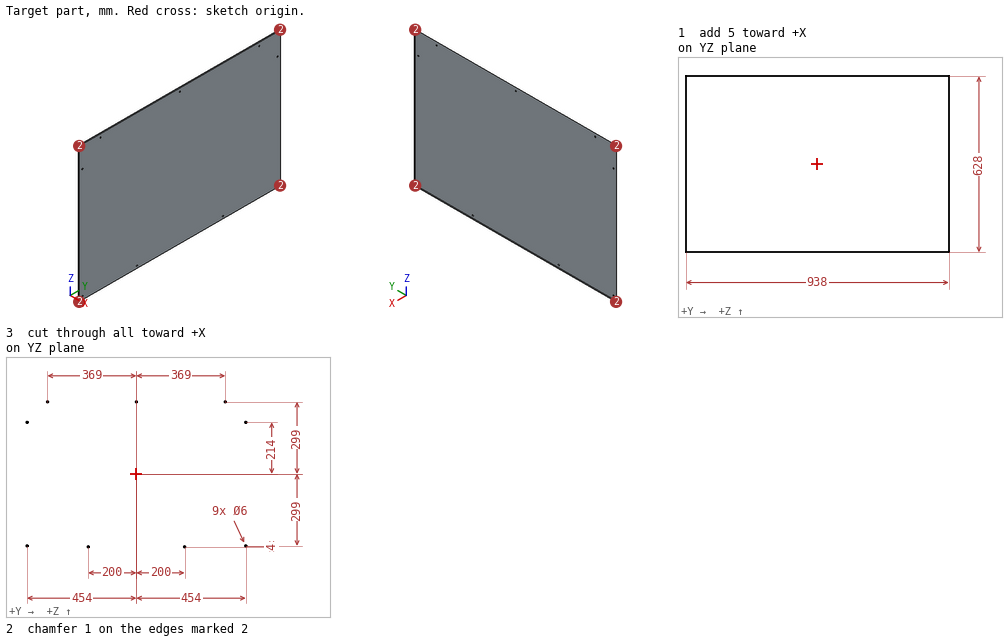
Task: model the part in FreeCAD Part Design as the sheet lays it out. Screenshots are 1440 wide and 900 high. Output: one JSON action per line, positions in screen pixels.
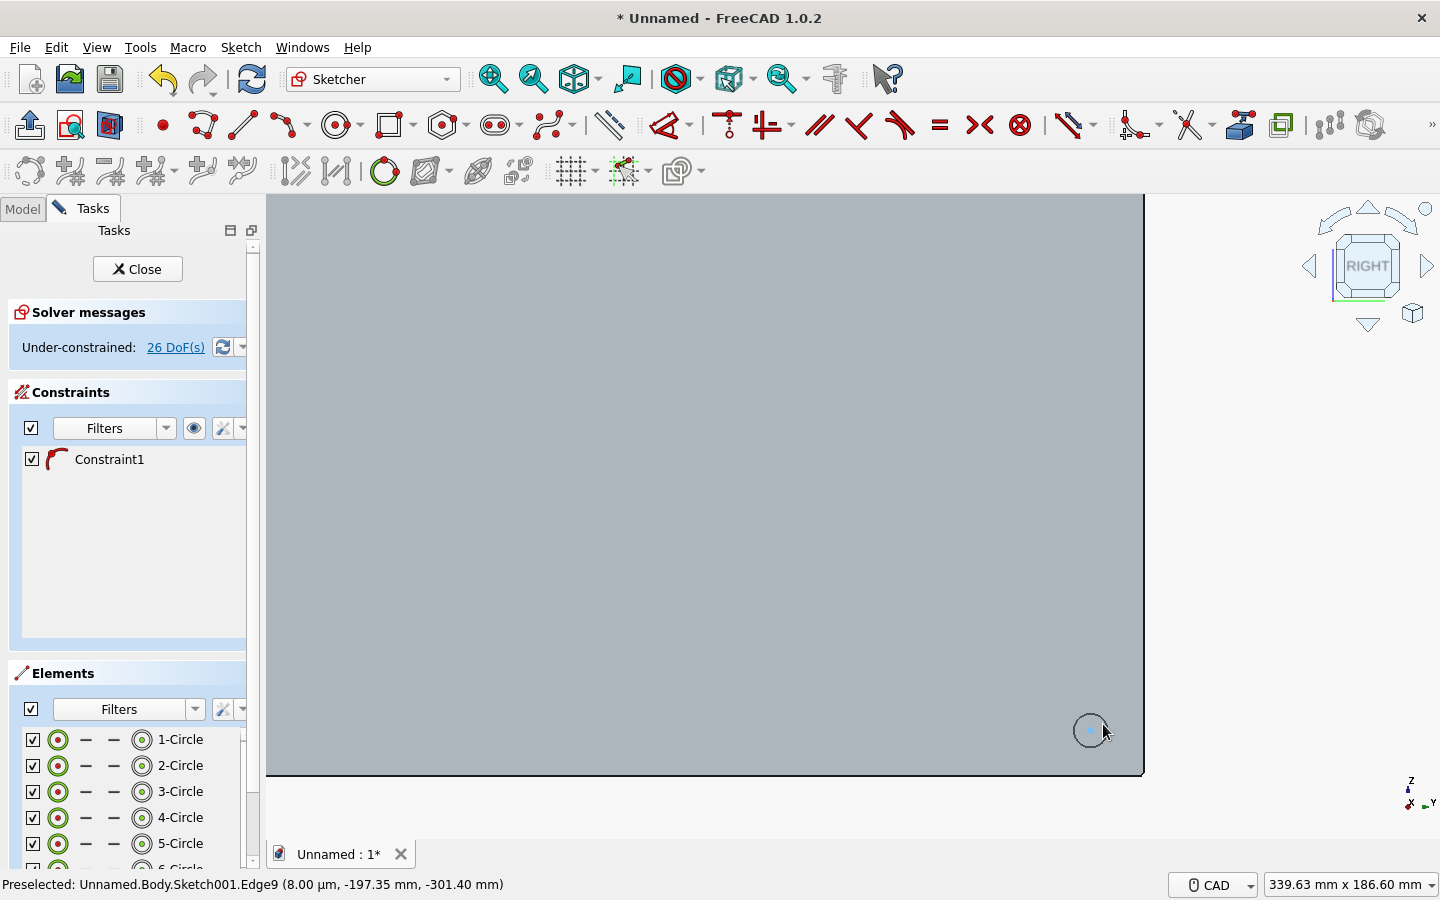
{"action": "left_click", "coordinate": [1103, 719]}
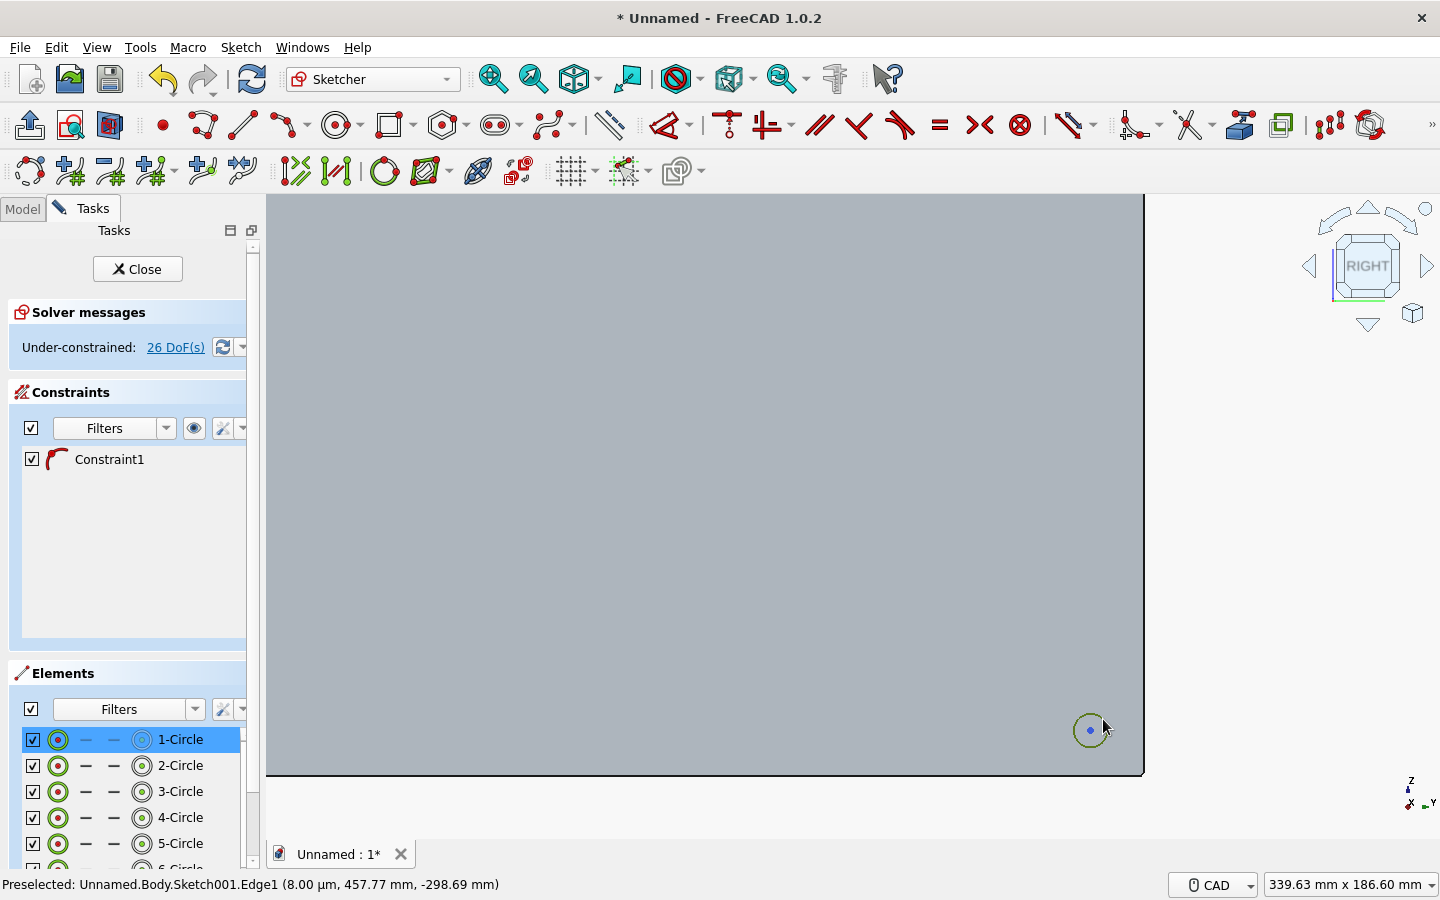
{"action": "scroll", "coordinate": [1104, 724], "scroll_direction": "down", "scroll_amount": 8}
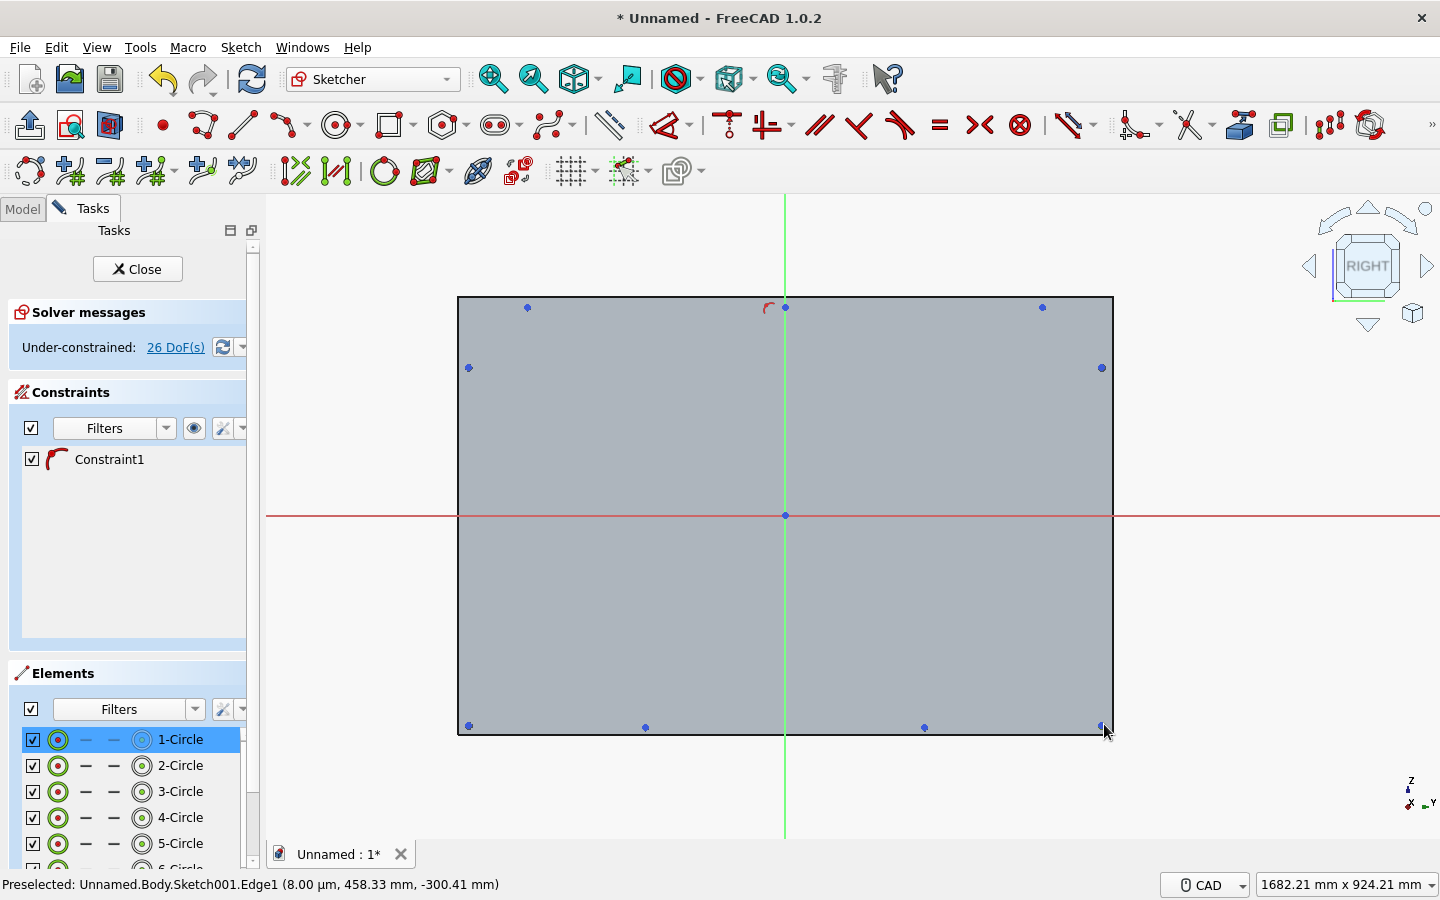
{"action": "scroll", "coordinate": [471, 724], "scroll_direction": "up", "scroll_amount": 8}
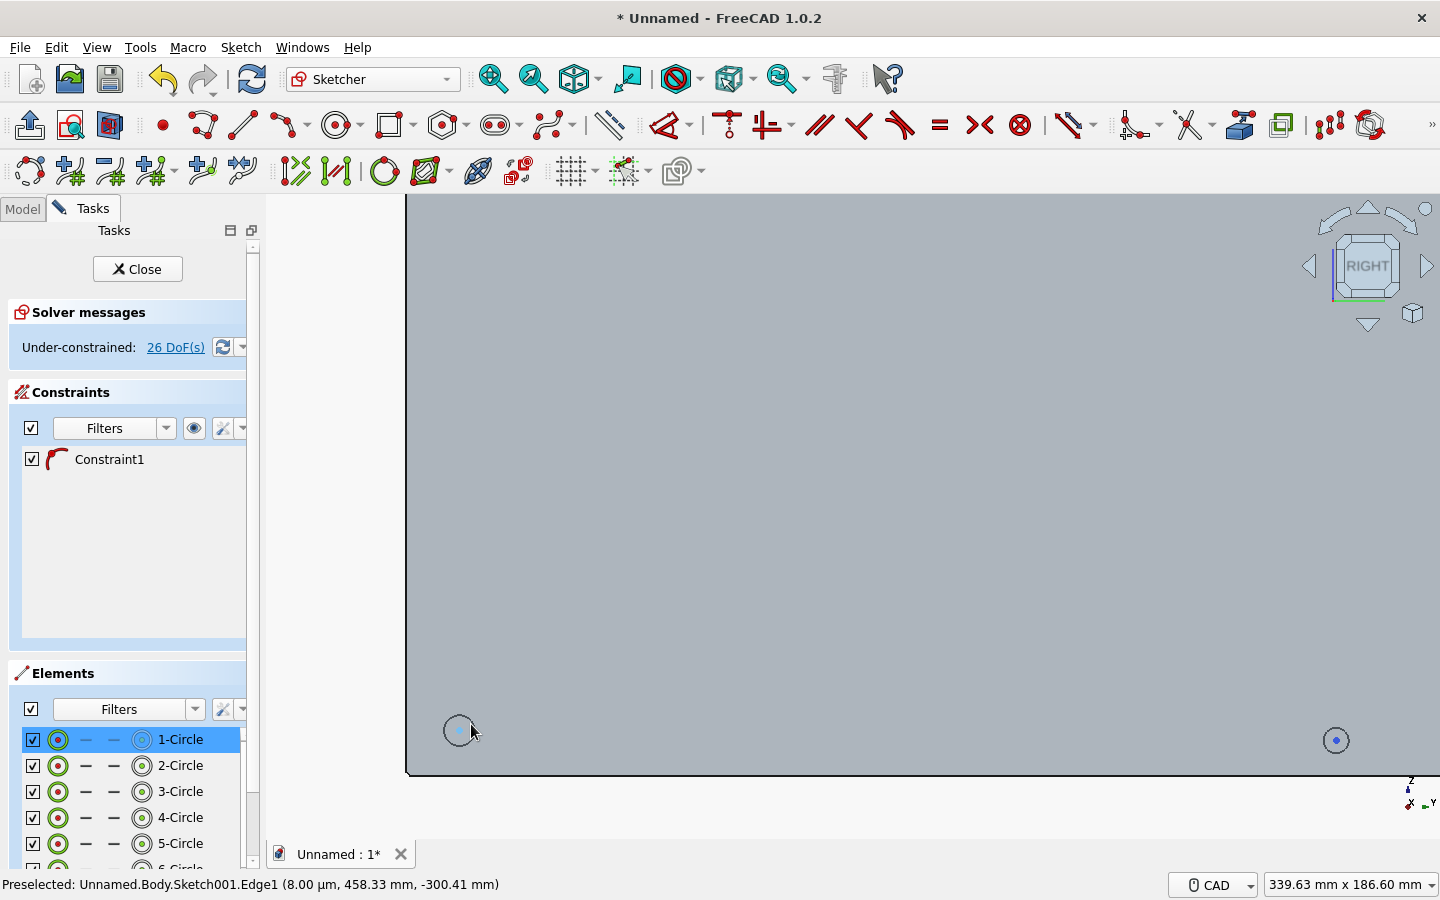
{"action": "left_click", "coordinate": [470, 720]}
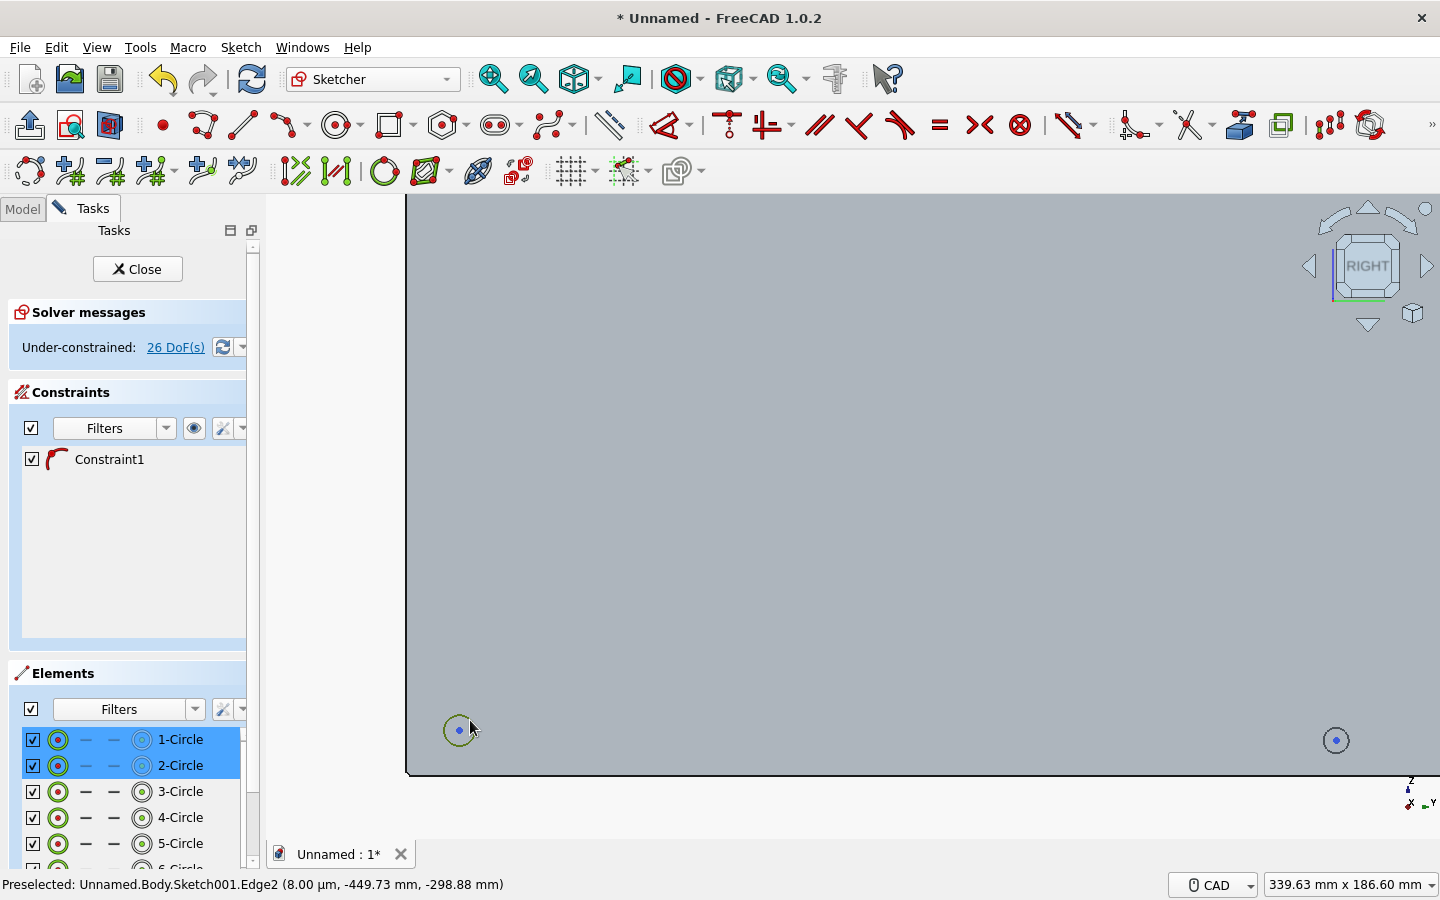
{"action": "scroll", "coordinate": [470, 724], "scroll_direction": "down", "scroll_amount": 8}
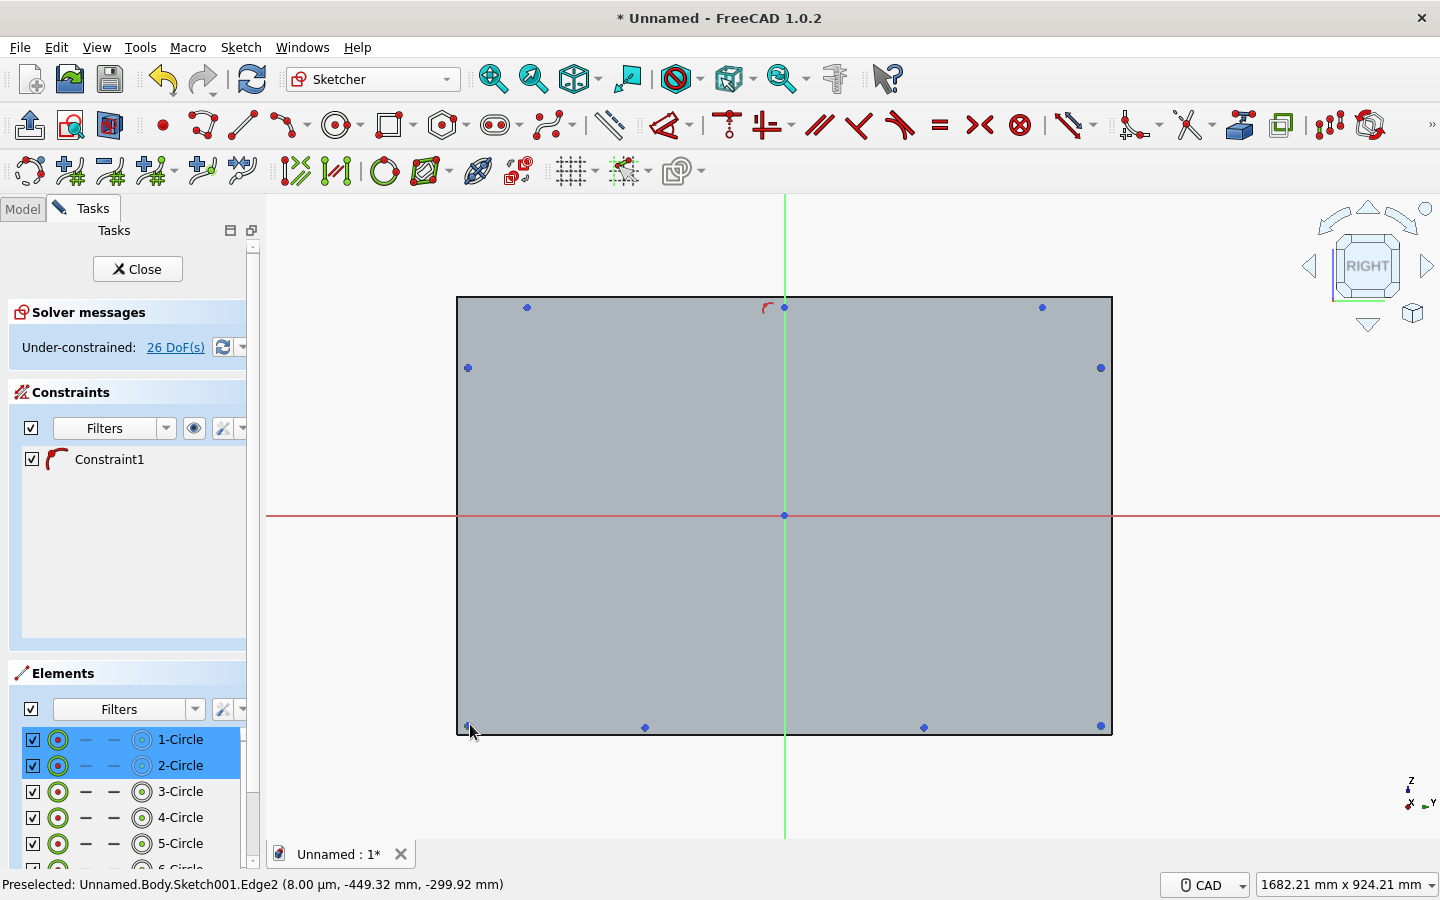
{"action": "scroll", "coordinate": [1103, 366], "scroll_direction": "up", "scroll_amount": 8}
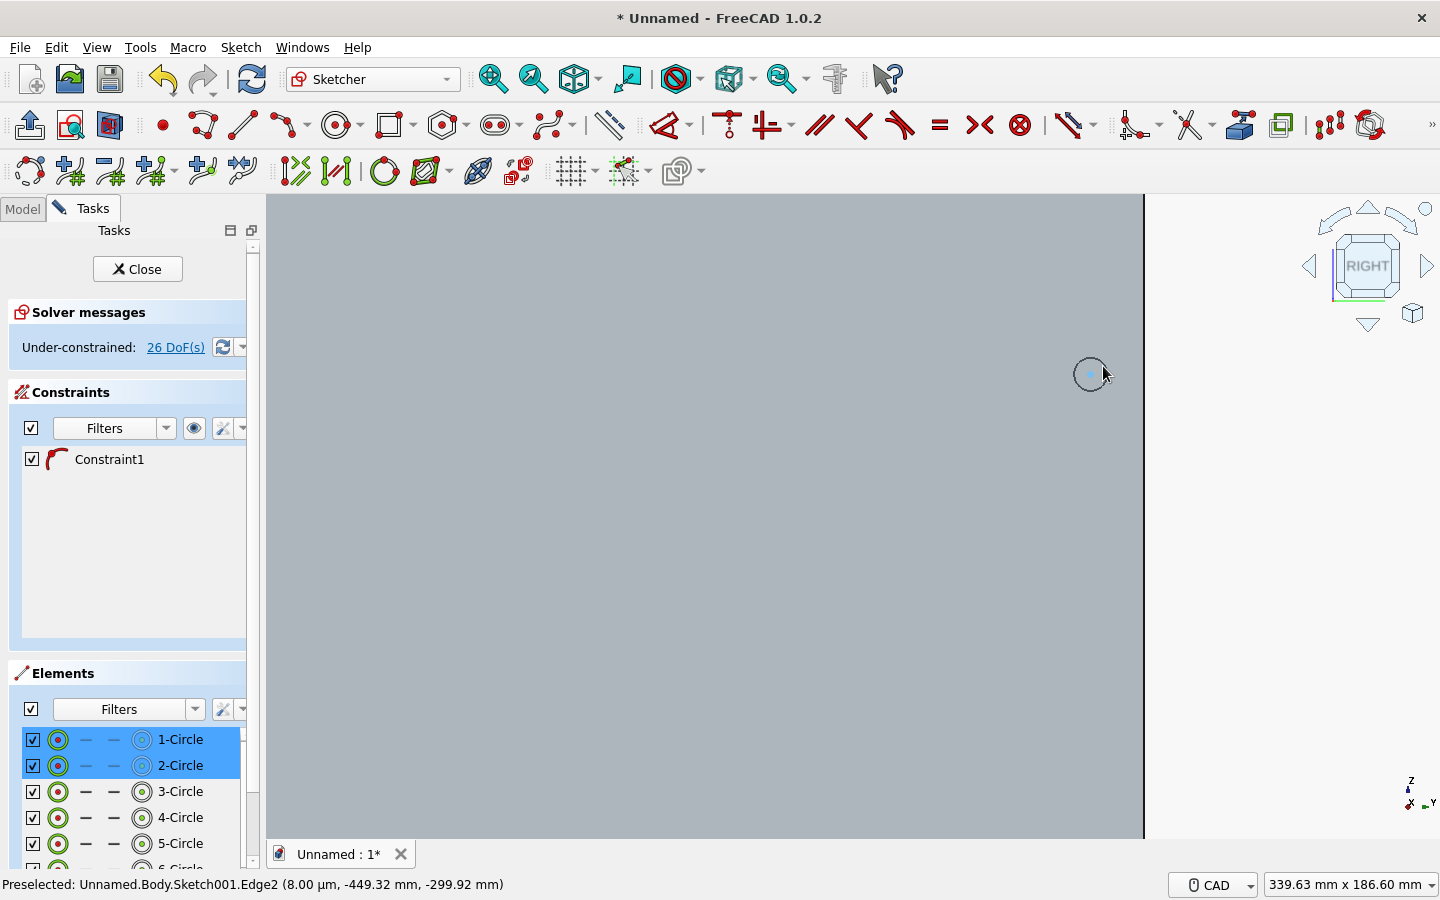
{"action": "left_click", "coordinate": [1102, 363]}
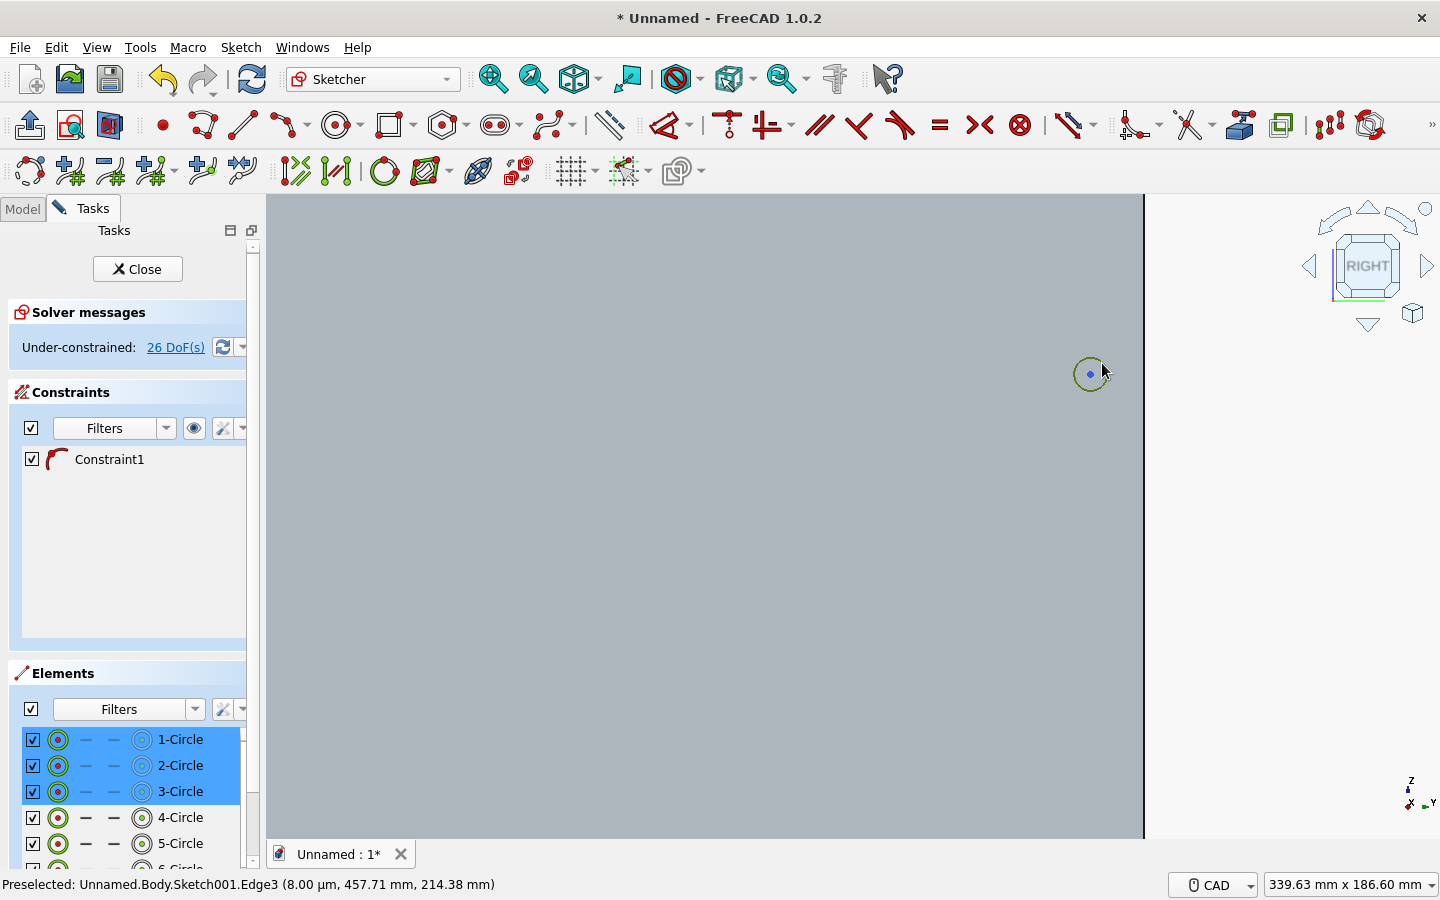
{"action": "scroll", "coordinate": [1104, 365], "scroll_direction": "down", "scroll_amount": 8}